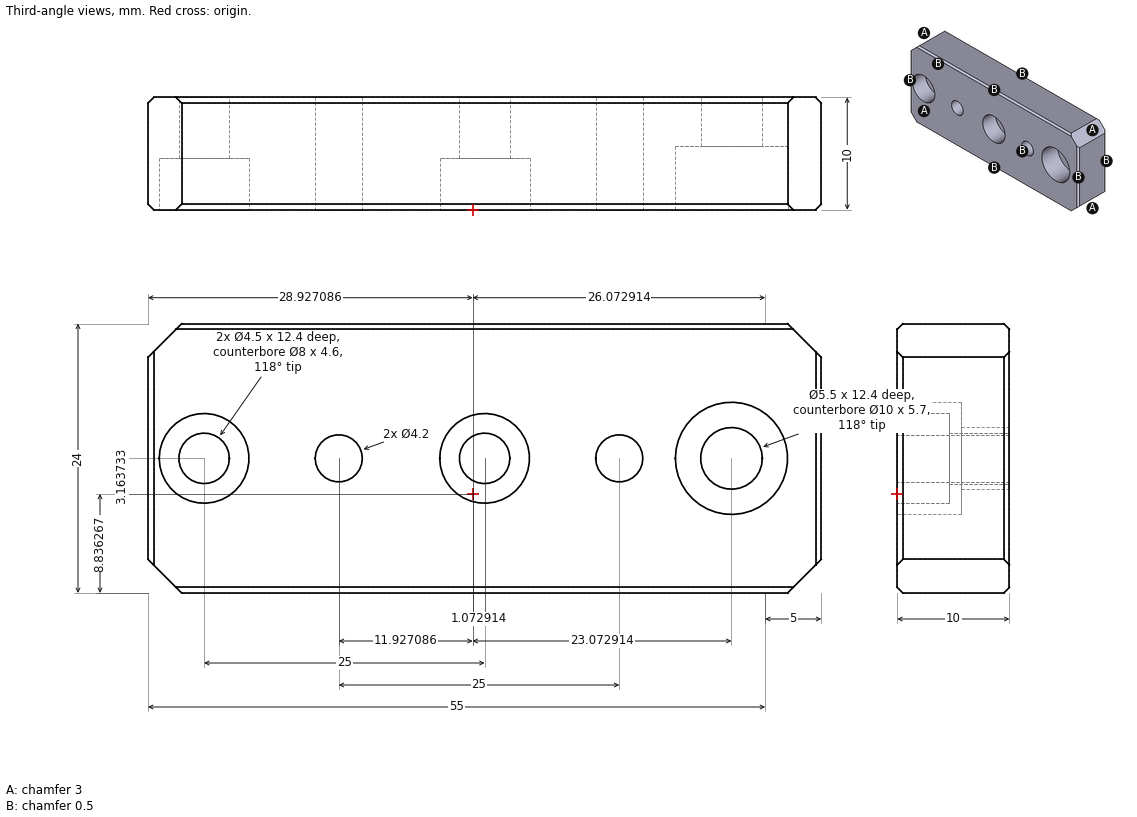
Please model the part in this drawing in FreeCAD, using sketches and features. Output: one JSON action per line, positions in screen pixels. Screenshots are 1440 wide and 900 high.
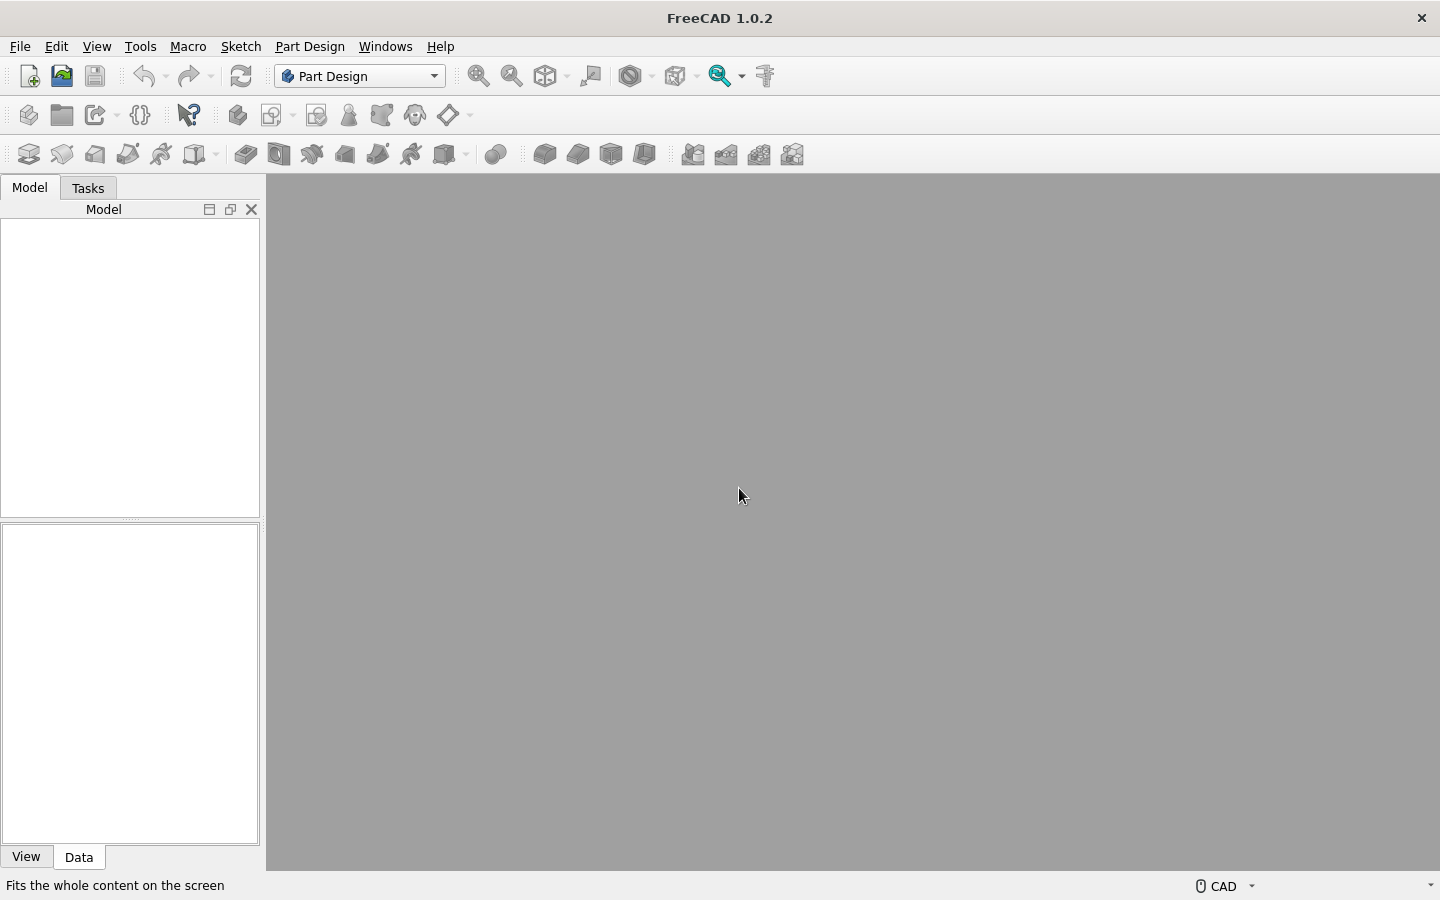
{"action": "left_click", "coordinate": [29, 76]}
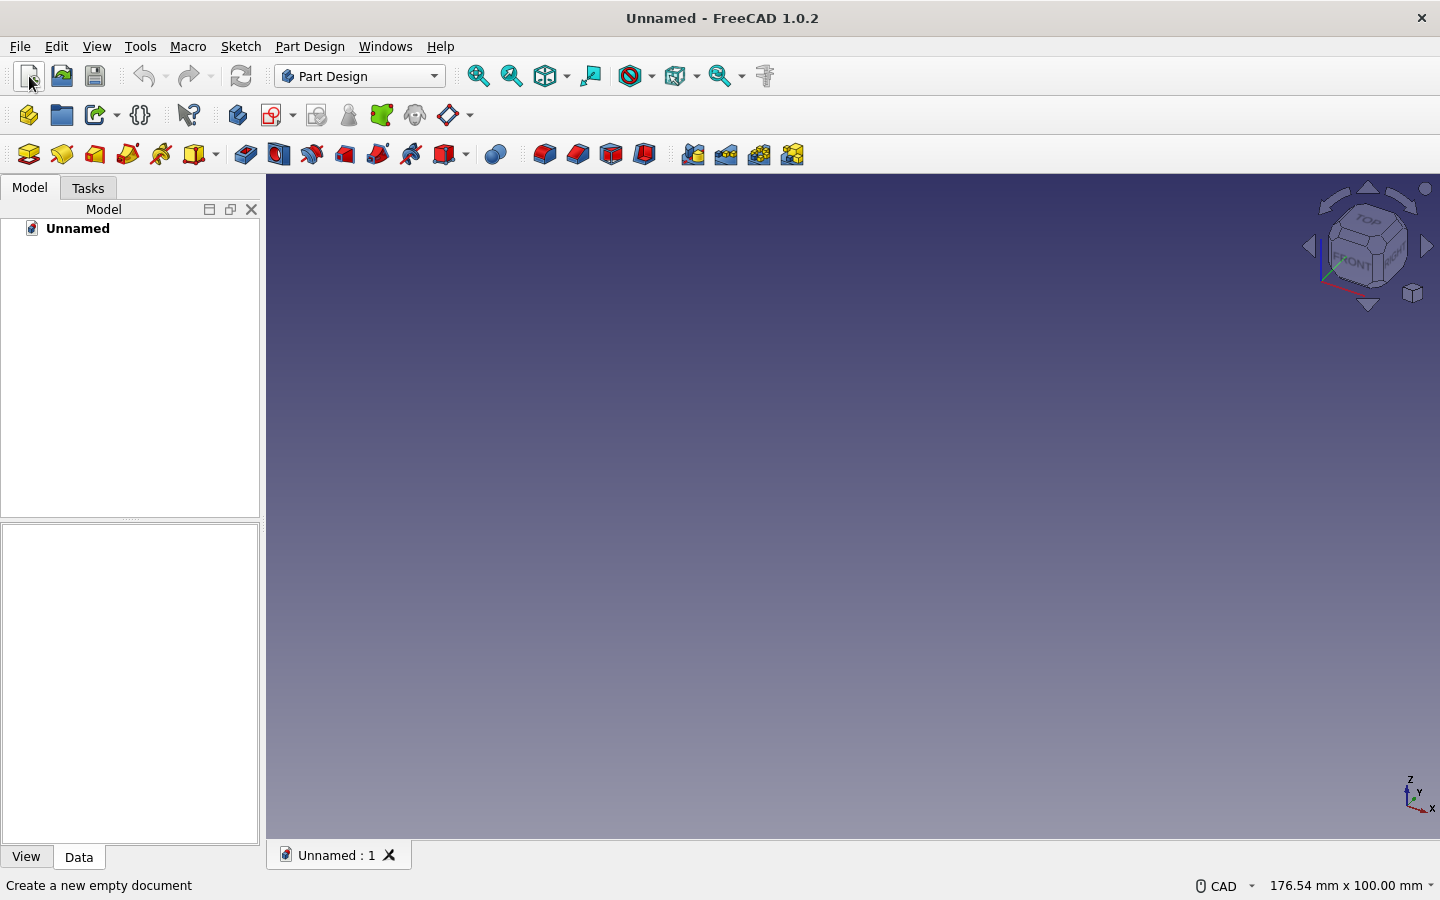
{"action": "left_click", "coordinate": [270, 116]}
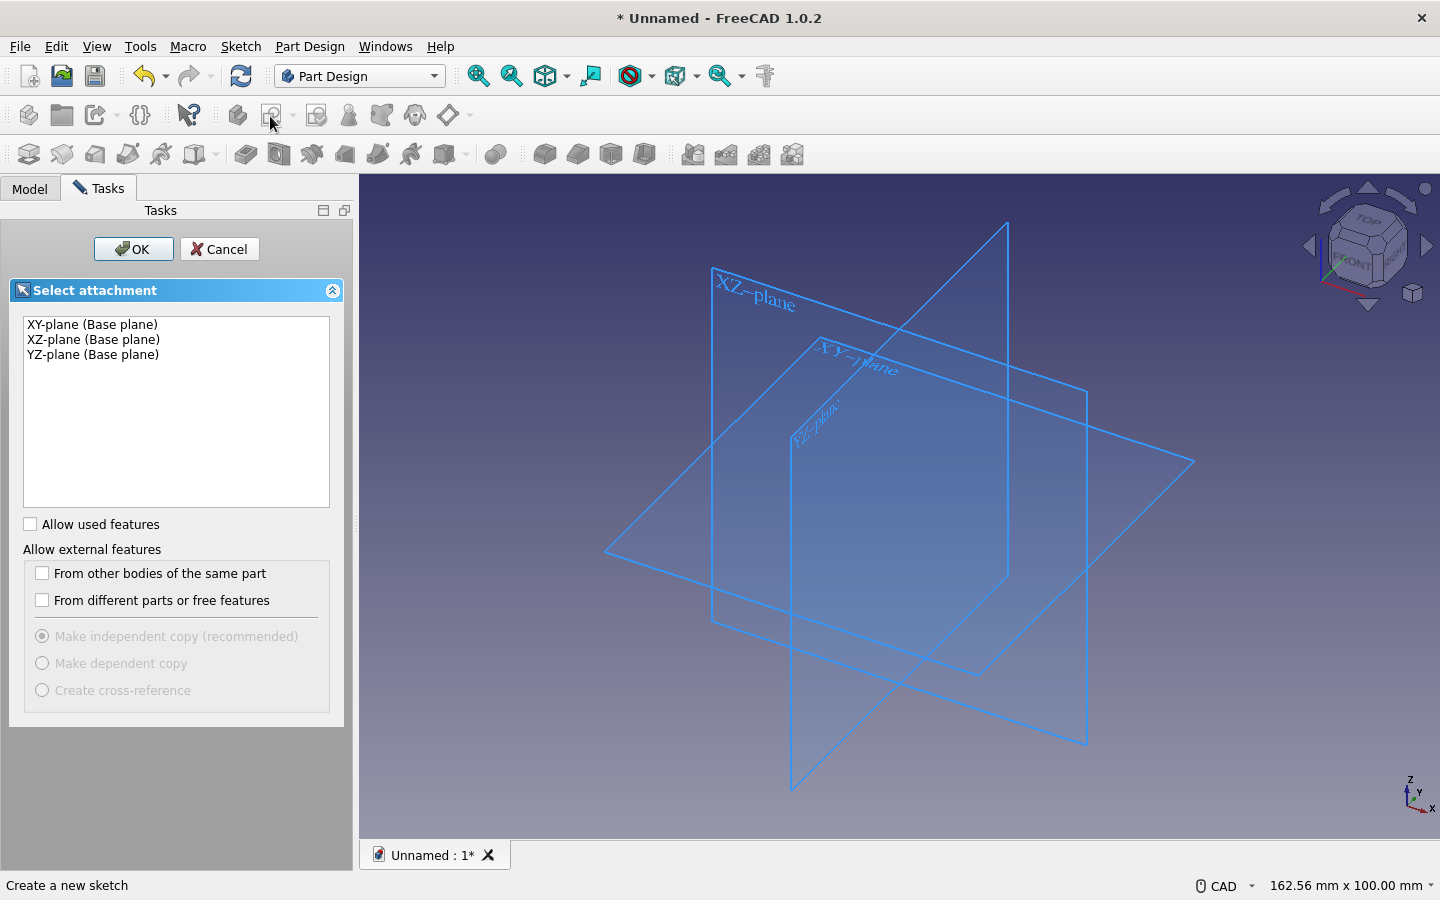
{"action": "left_click", "coordinate": [84, 340]}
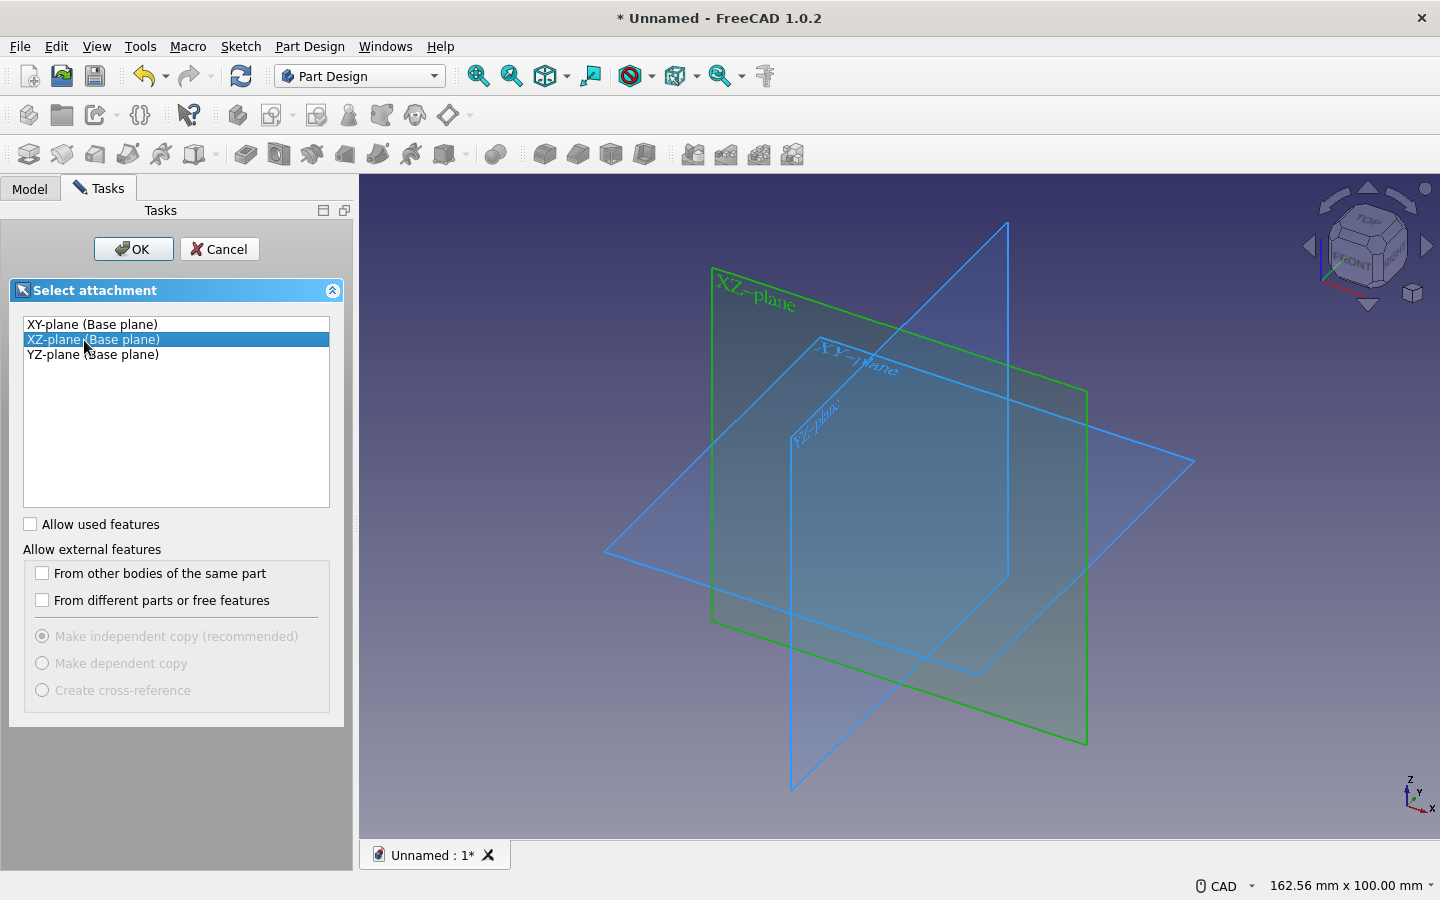
{"action": "left_click", "coordinate": [134, 249]}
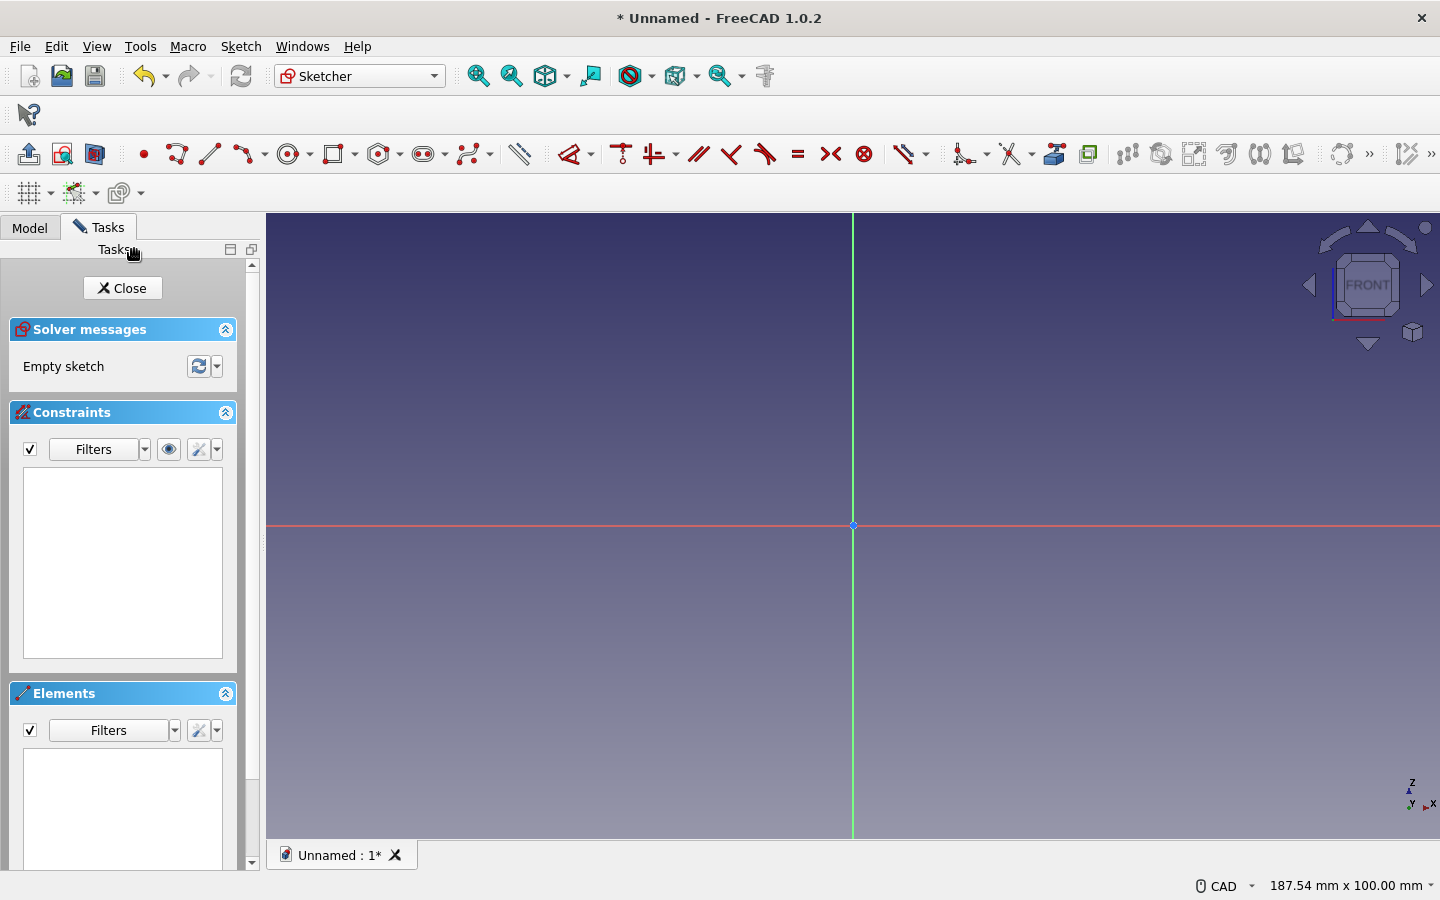
{"action": "scroll", "coordinate": [917, 482], "scroll_direction": "up", "scroll_amount": 3}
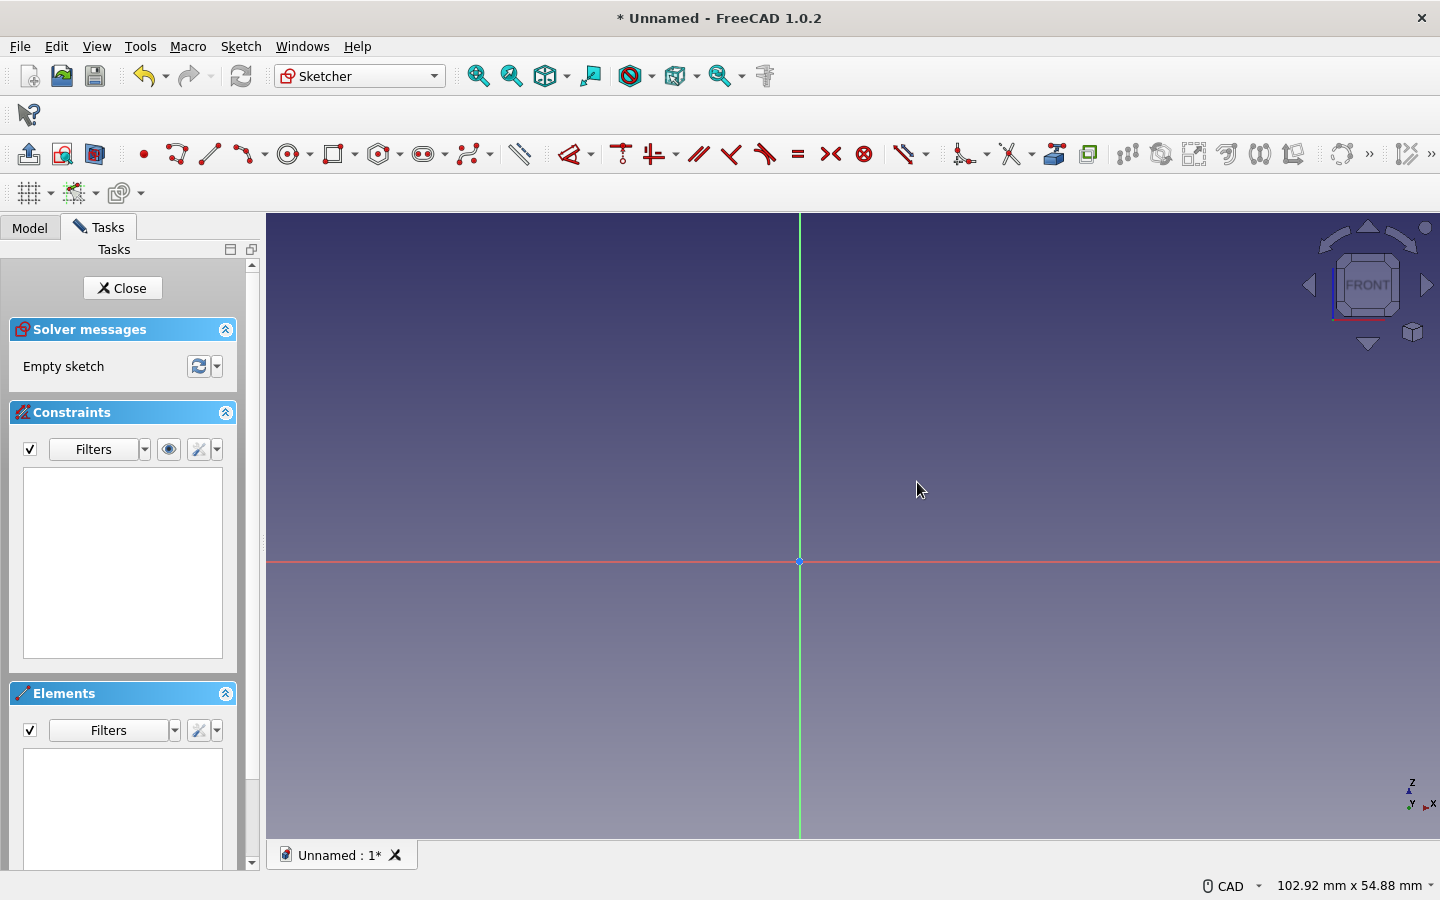
{"action": "key", "text": "g r"}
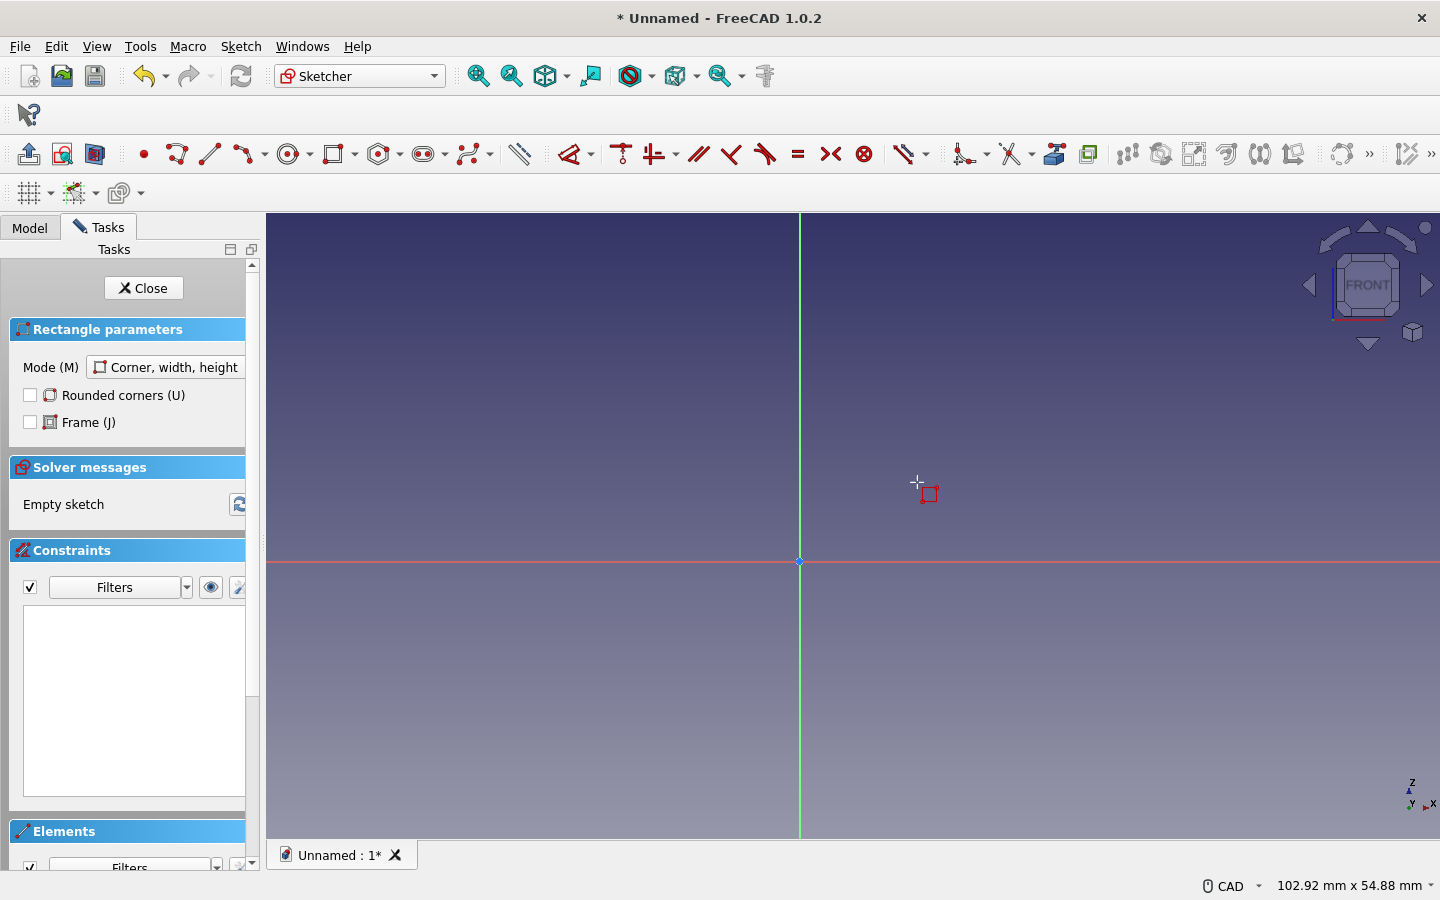
{"action": "left_click", "coordinate": [470, 389]}
{"action": "left_click", "coordinate": [1097, 663]}
{"action": "key", "text": "Escape"}